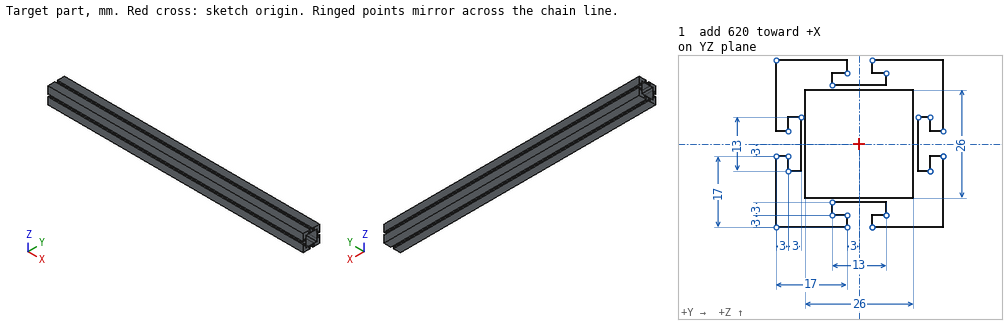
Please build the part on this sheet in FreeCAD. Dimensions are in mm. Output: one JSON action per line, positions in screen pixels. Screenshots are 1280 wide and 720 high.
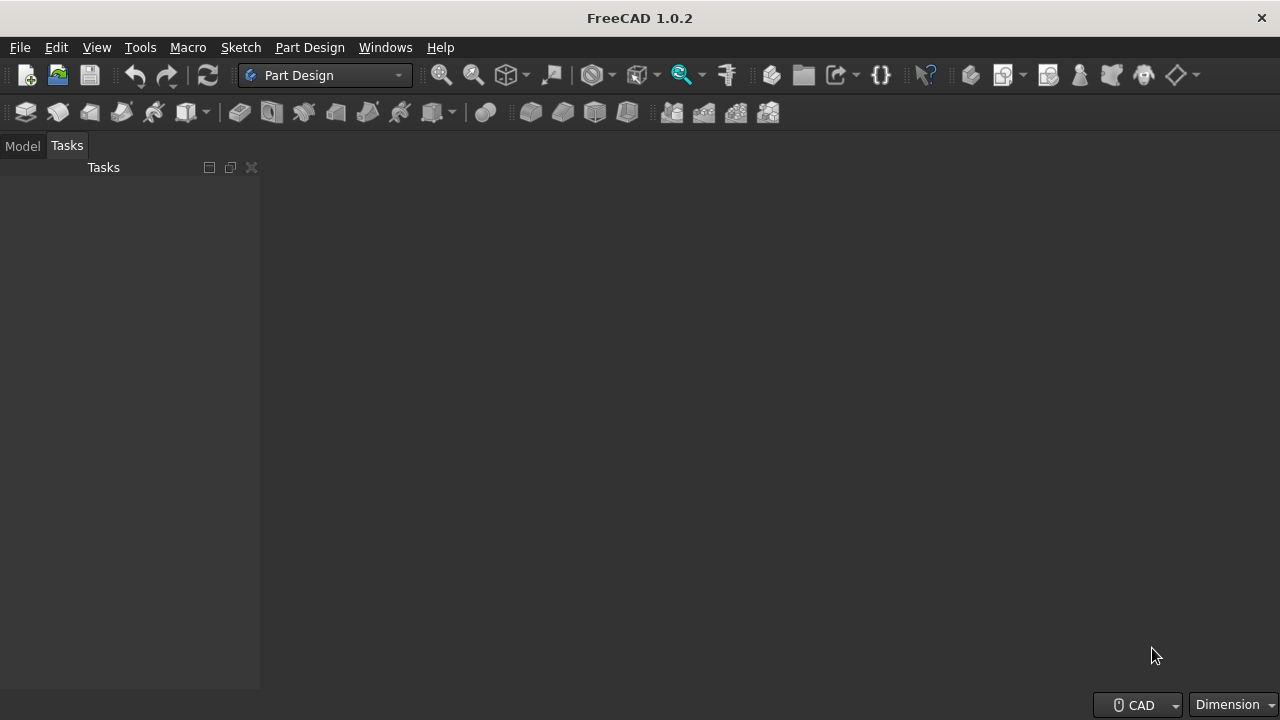
{"action": "key", "text": "ctrl+n"}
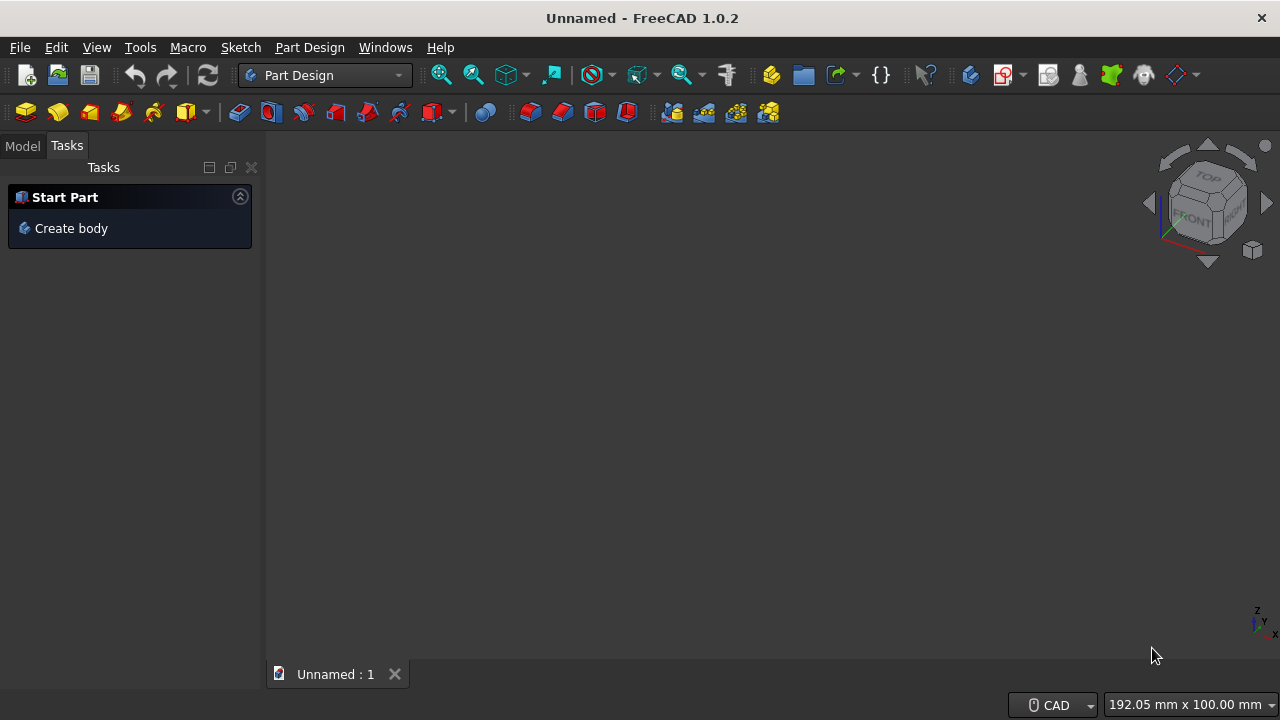
{"action": "left_click", "coordinate": [1004, 76]}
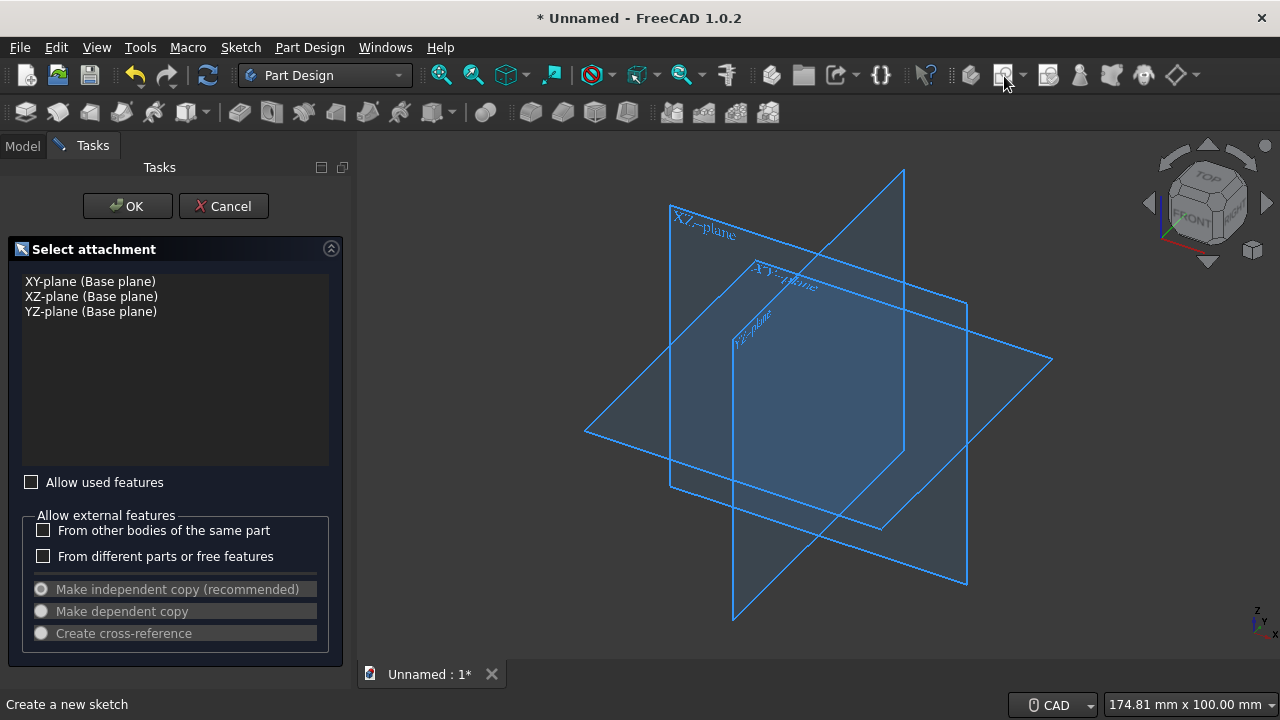
{"action": "left_click", "coordinate": [82, 312]}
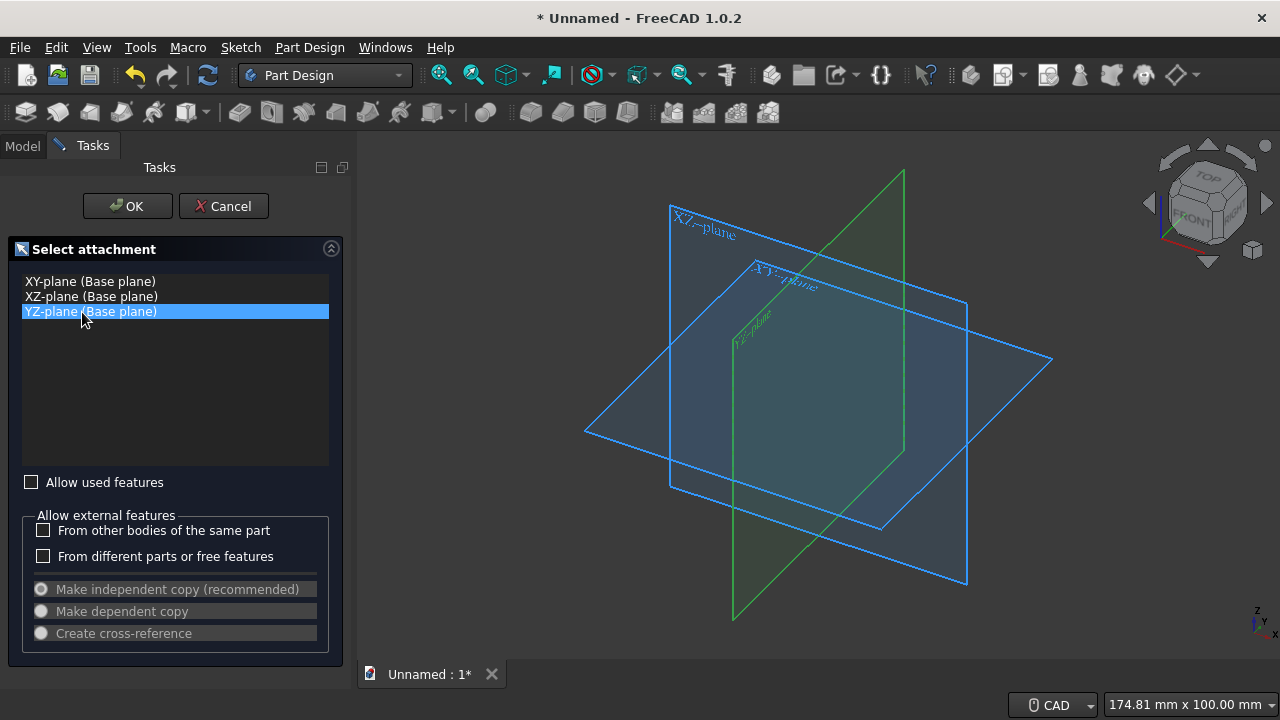
{"action": "left_click", "coordinate": [128, 206]}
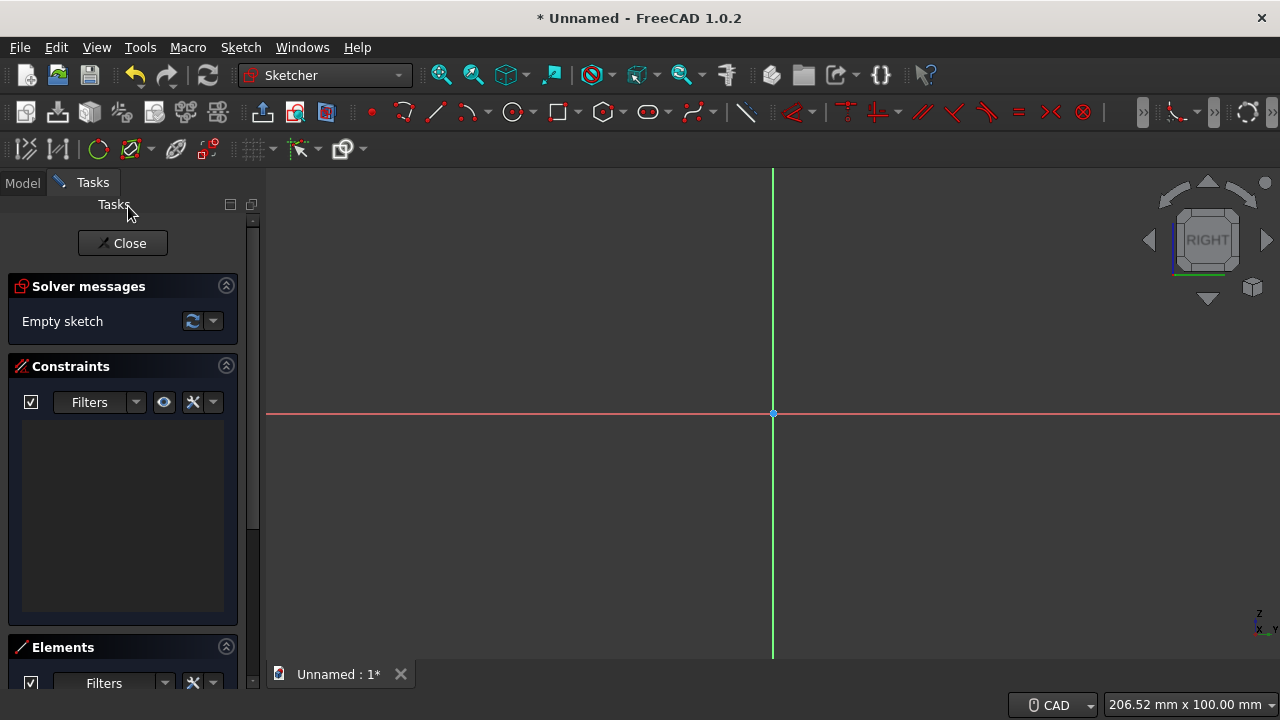
{"action": "scroll", "coordinate": [912, 413], "scroll_direction": "up", "scroll_amount": 2}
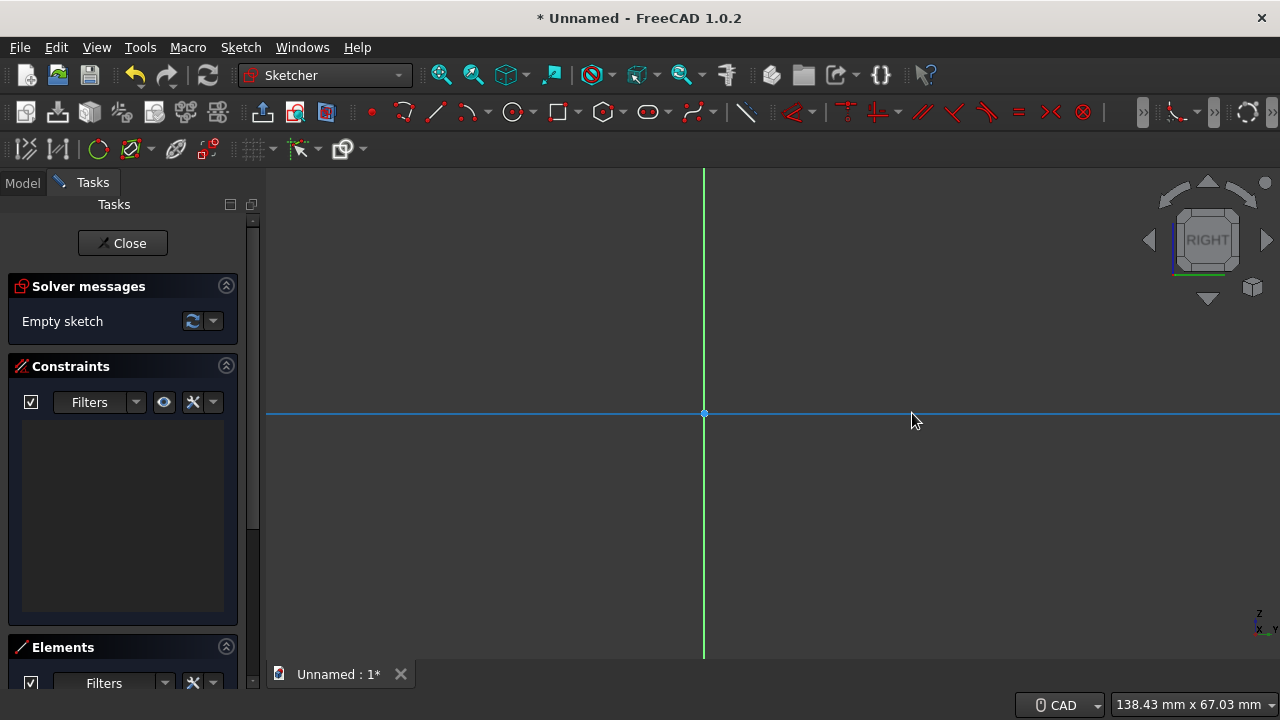
{"action": "left_click", "coordinate": [404, 112]}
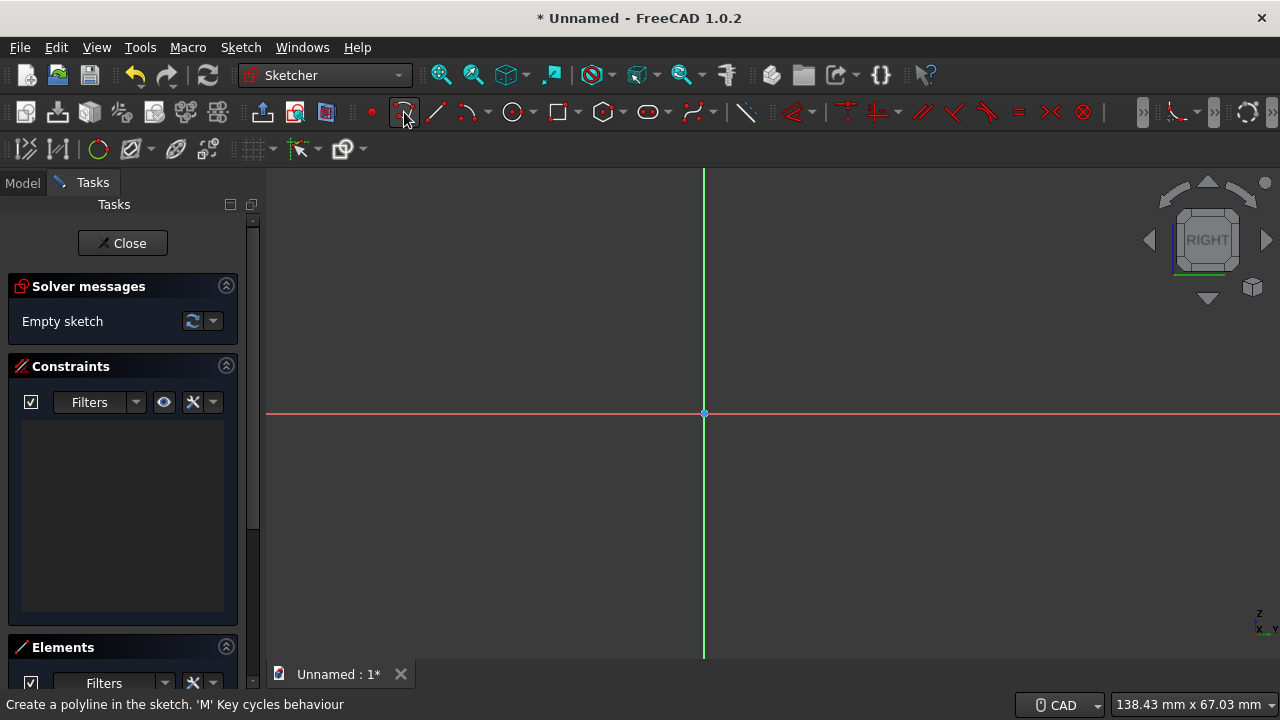
{"action": "left_click", "coordinate": [602, 366]}
{"action": "left_click", "coordinate": [602, 461]}
{"action": "left_click", "coordinate": [580, 461]}
{"action": "left_click", "coordinate": [580, 435]}
{"action": "left_click", "coordinate": [558, 435]}
{"action": "left_click", "coordinate": [558, 560]}
{"action": "left_click", "coordinate": [682, 560]}
{"action": "left_click", "coordinate": [682, 538]}
{"action": "left_click", "coordinate": [657, 538]}
{"action": "left_click", "coordinate": [657, 516]}
{"action": "left_click", "coordinate": [752, 516]}
{"action": "left_click", "coordinate": [752, 538]}
{"action": "left_click", "coordinate": [726, 538]}
{"action": "left_click", "coordinate": [726, 560]}
{"action": "left_click", "coordinate": [851, 560]}
{"action": "left_click", "coordinate": [851, 435]}
{"action": "left_click", "coordinate": [829, 435]}
{"action": "left_click", "coordinate": [829, 461]}
{"action": "left_click", "coordinate": [807, 461]}
{"action": "left_click", "coordinate": [807, 366]}
{"action": "left_click", "coordinate": [829, 366]}
{"action": "left_click", "coordinate": [829, 392]}
{"action": "left_click", "coordinate": [851, 392]}
{"action": "left_click", "coordinate": [851, 267]}
{"action": "left_click", "coordinate": [726, 267]}
{"action": "left_click", "coordinate": [726, 289]}
{"action": "left_click", "coordinate": [752, 289]}
{"action": "left_click", "coordinate": [752, 311]}
{"action": "left_click", "coordinate": [657, 311]}
{"action": "left_click", "coordinate": [657, 289]}
{"action": "left_click", "coordinate": [682, 289]}
{"action": "left_click", "coordinate": [682, 267]}
{"action": "left_click", "coordinate": [558, 267]}
{"action": "left_click", "coordinate": [558, 392]}
{"action": "left_click", "coordinate": [580, 392]}
{"action": "left_click", "coordinate": [580, 366]}
{"action": "left_click", "coordinate": [602, 367]}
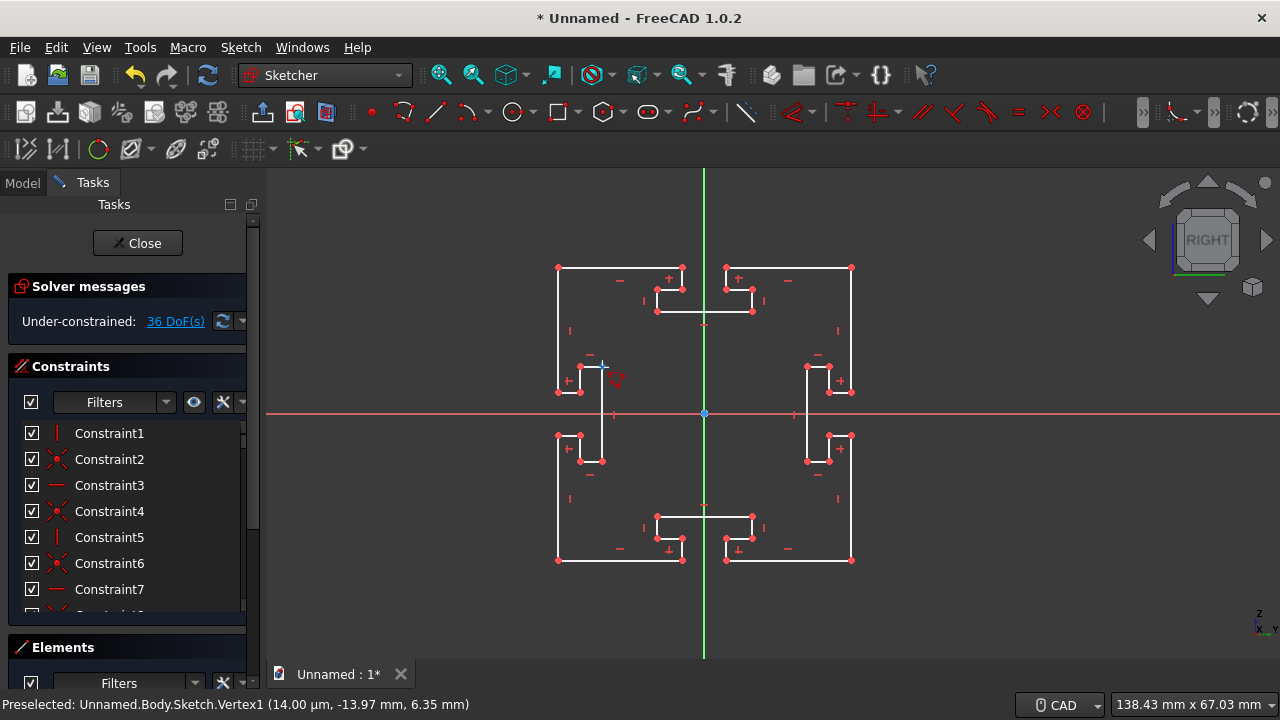
{"action": "key", "text": "g v"}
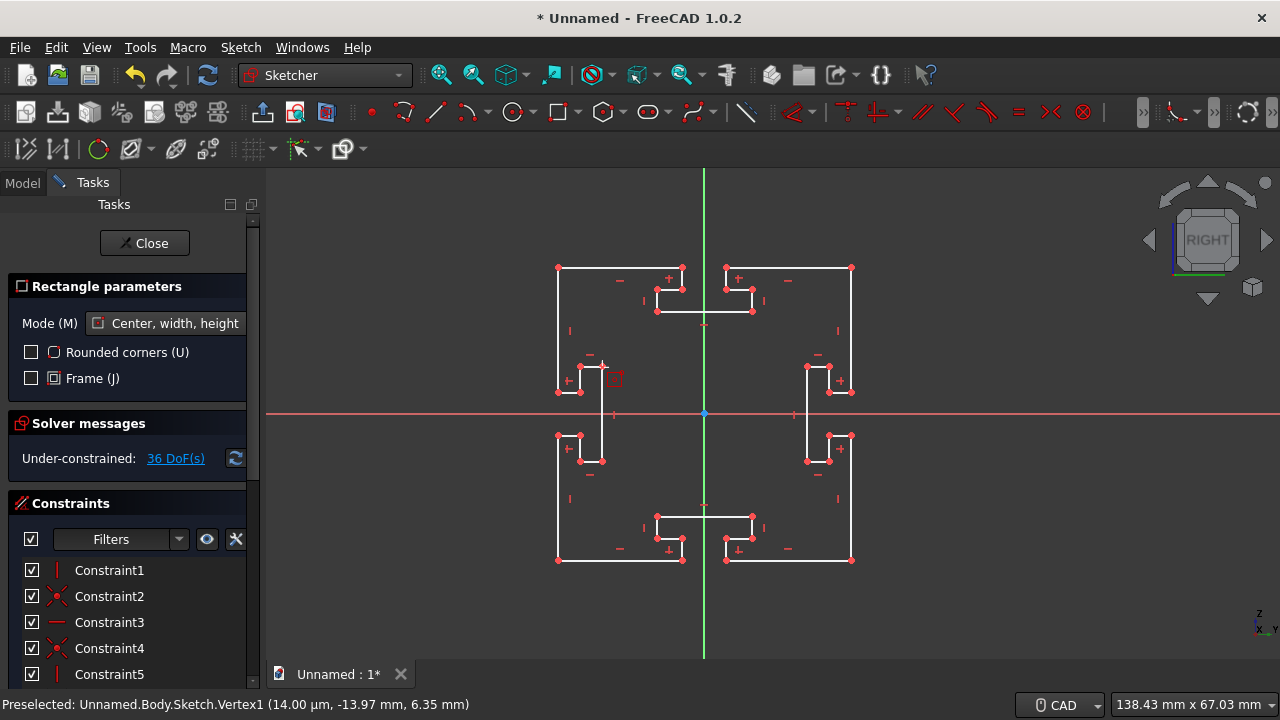
{"action": "left_click", "coordinate": [704, 414]}
{"action": "mouse_move", "coordinate": [800, 318]}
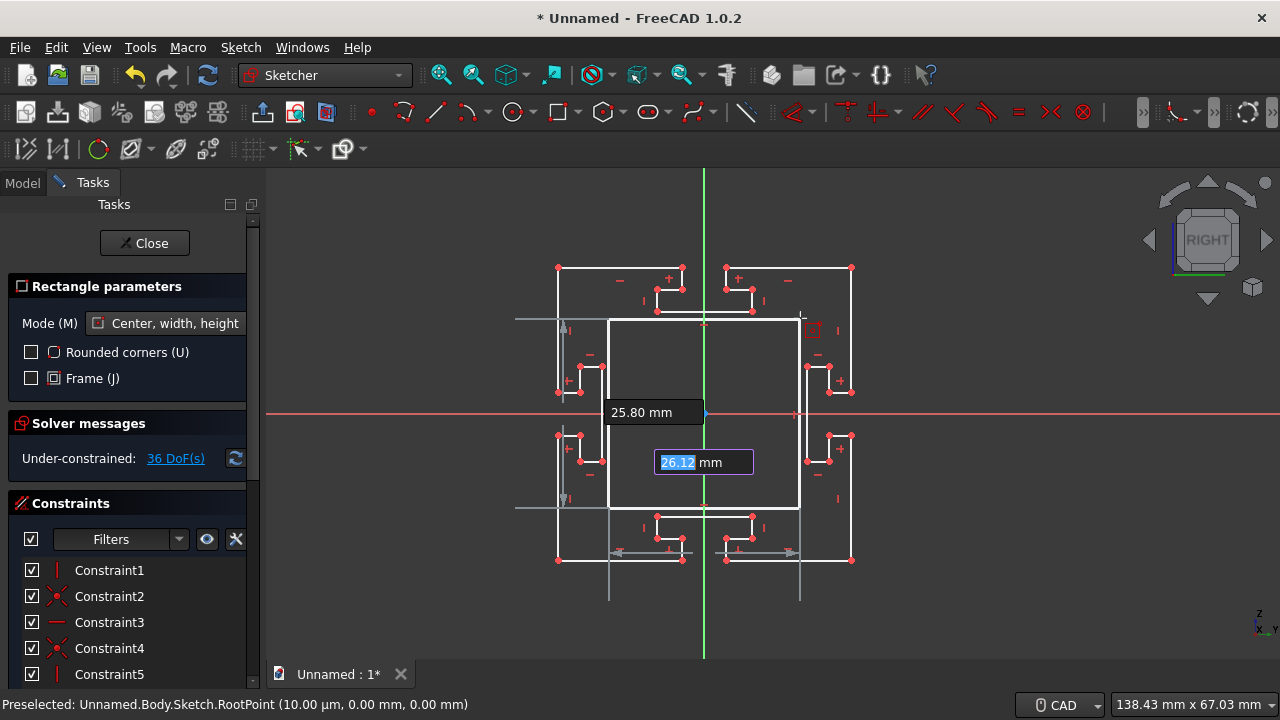
{"action": "type", "text": "26"}
{"action": "key", "text": "Tab"}
{"action": "type", "text": "26"}
{"action": "key", "text": "Return"}
{"action": "key", "text": "Escape"}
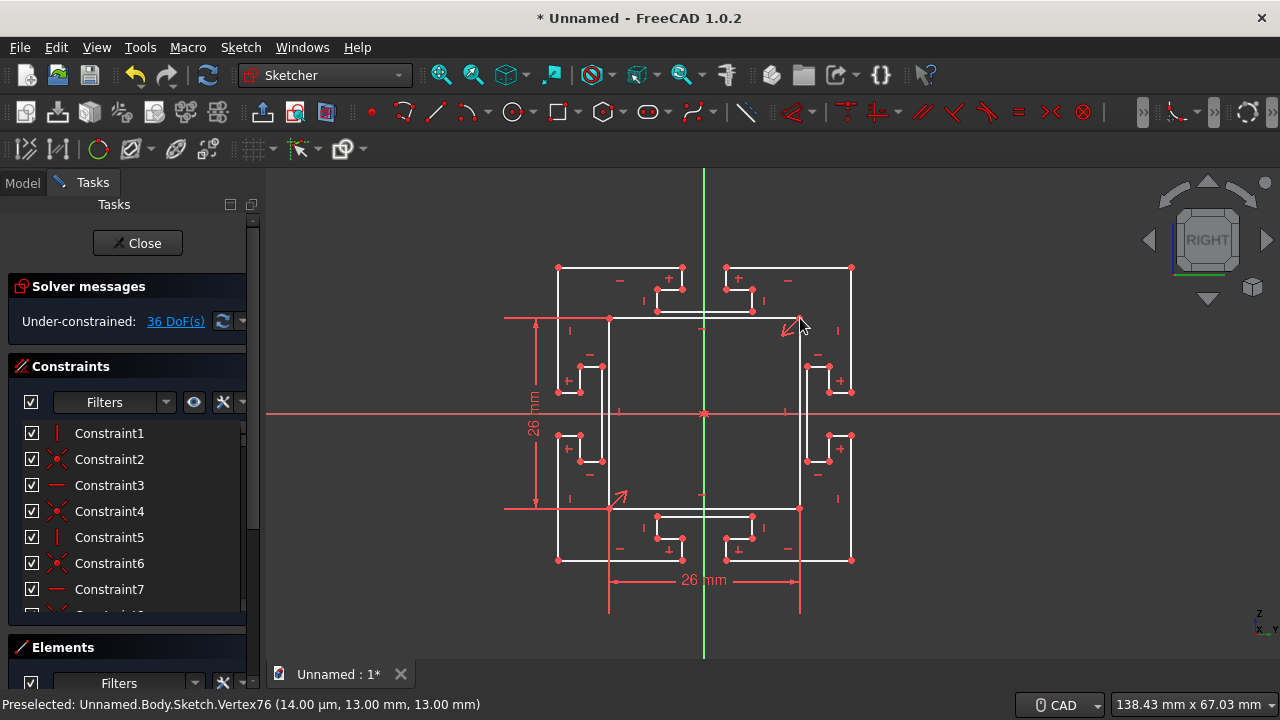
{"action": "left_click", "coordinate": [657, 539]}